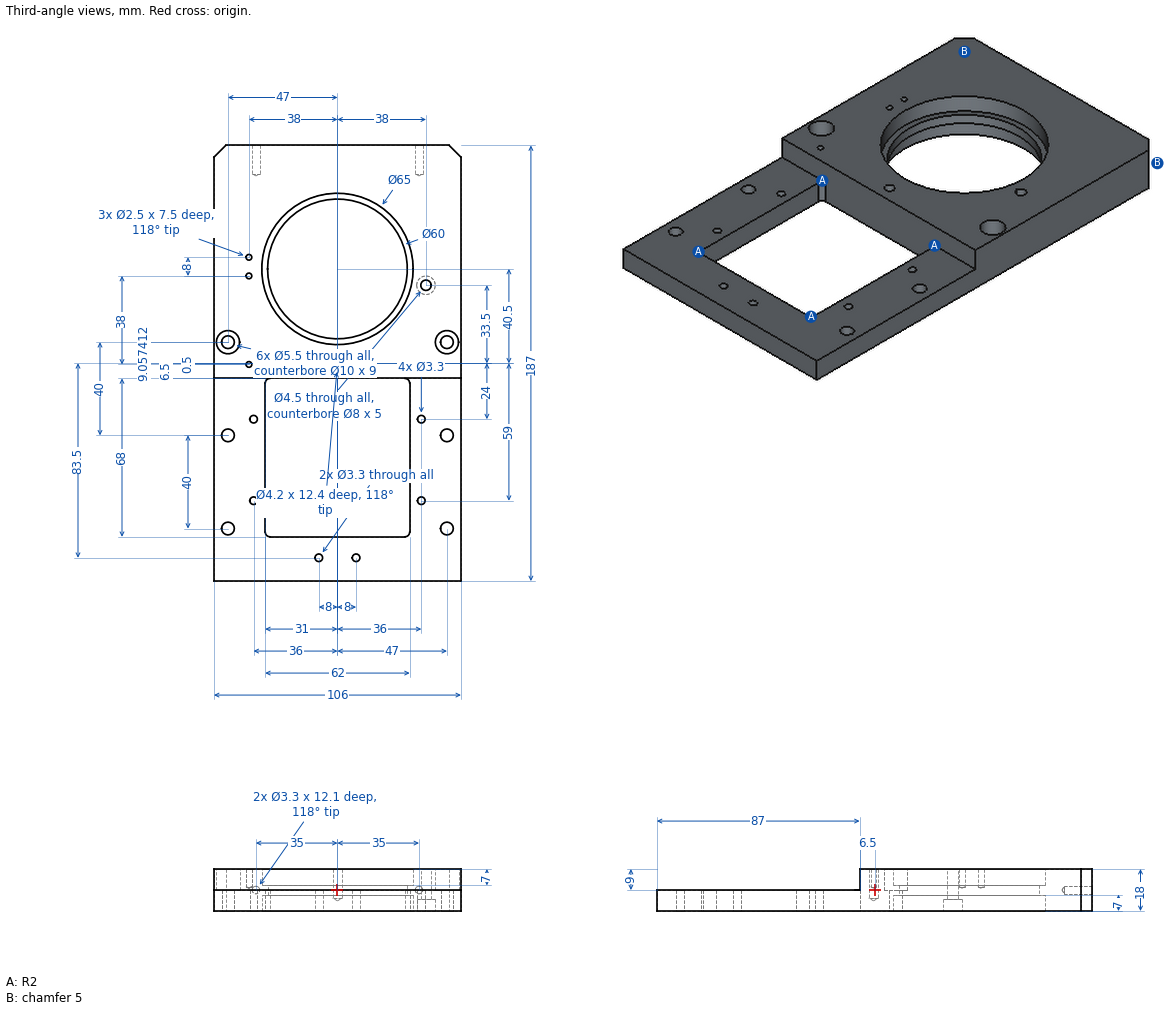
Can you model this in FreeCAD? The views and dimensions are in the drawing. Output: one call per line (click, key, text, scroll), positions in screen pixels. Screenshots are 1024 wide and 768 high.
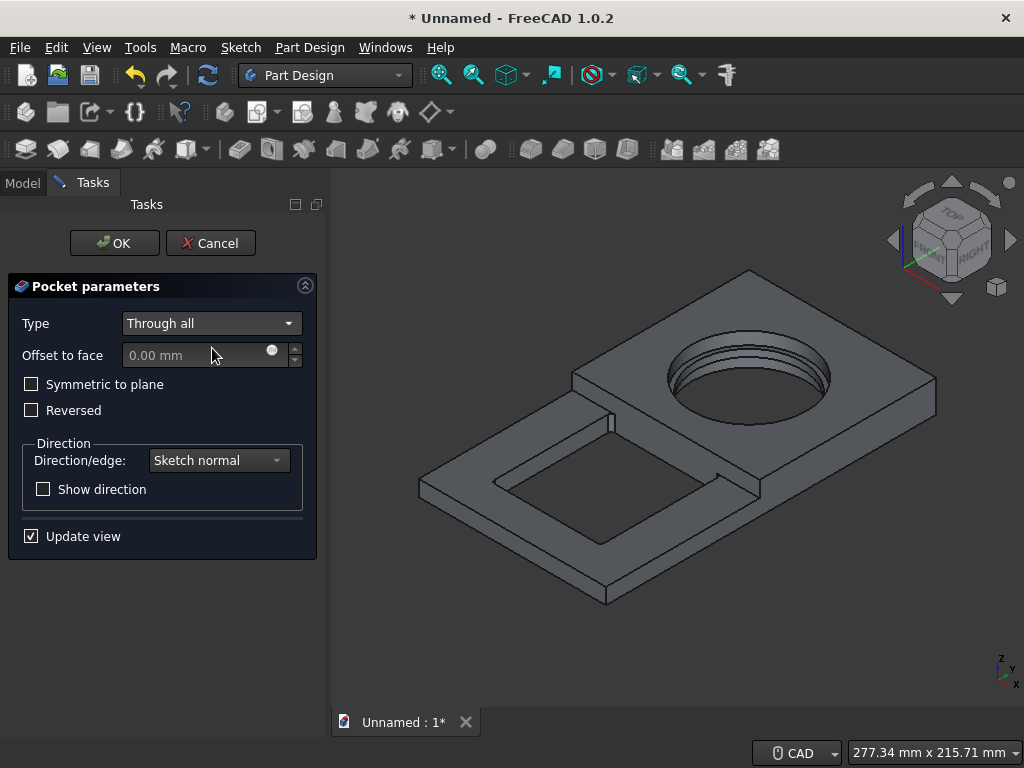
click(115, 243)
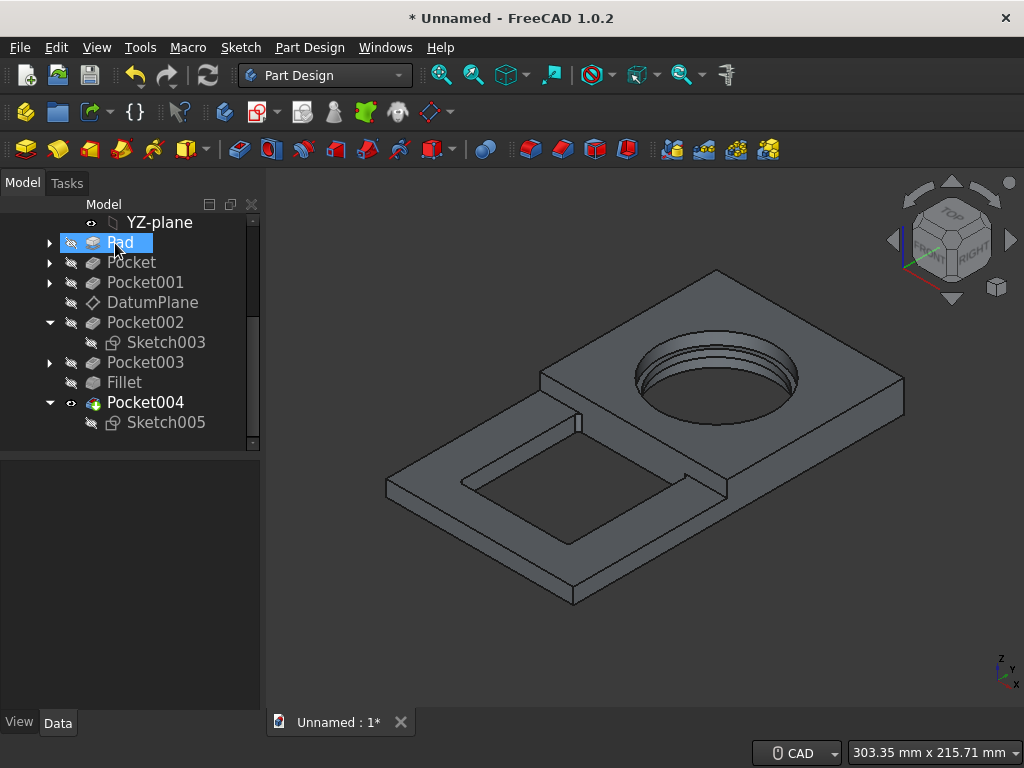
click(258, 112)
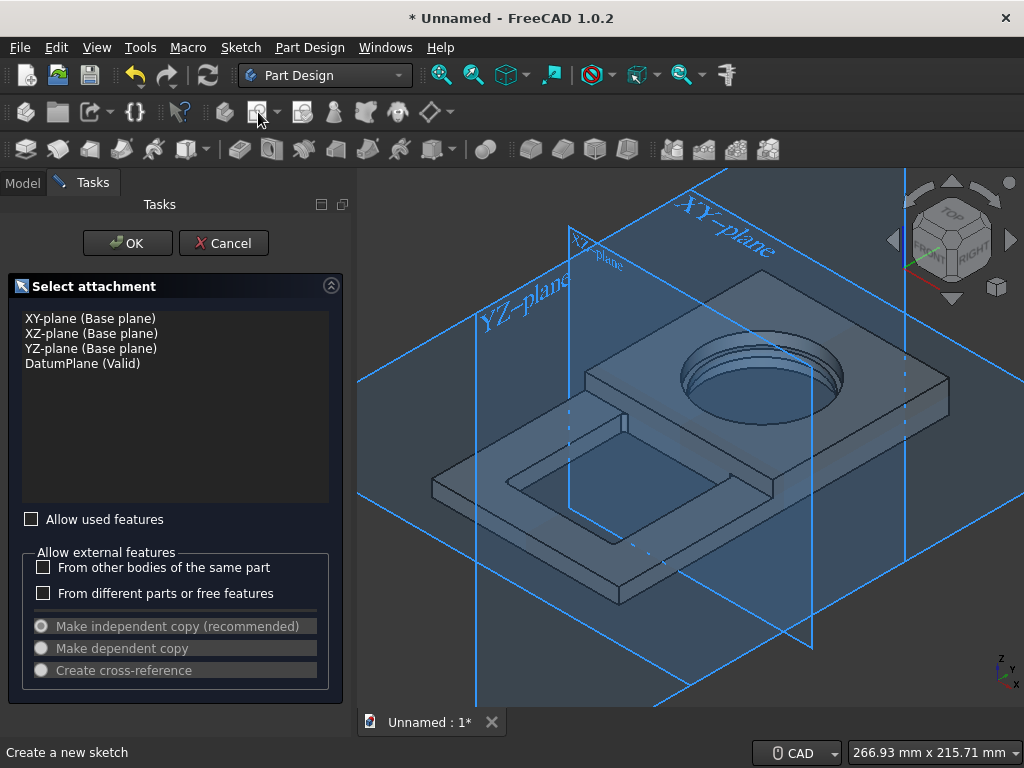
click(82, 318)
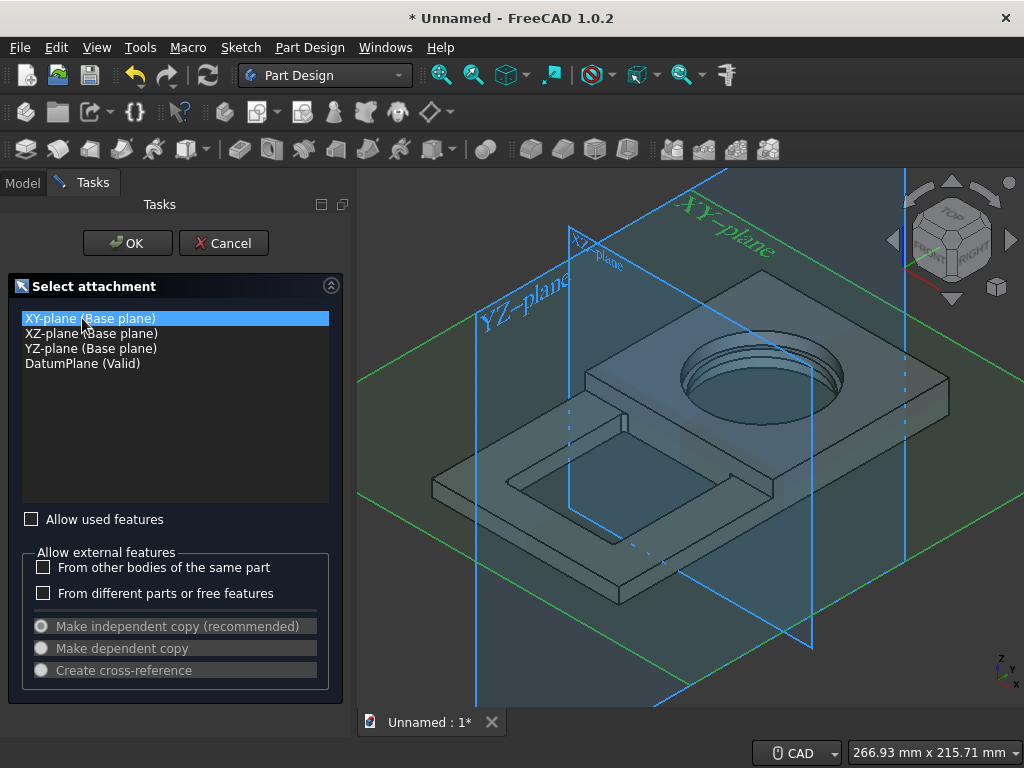
click(128, 243)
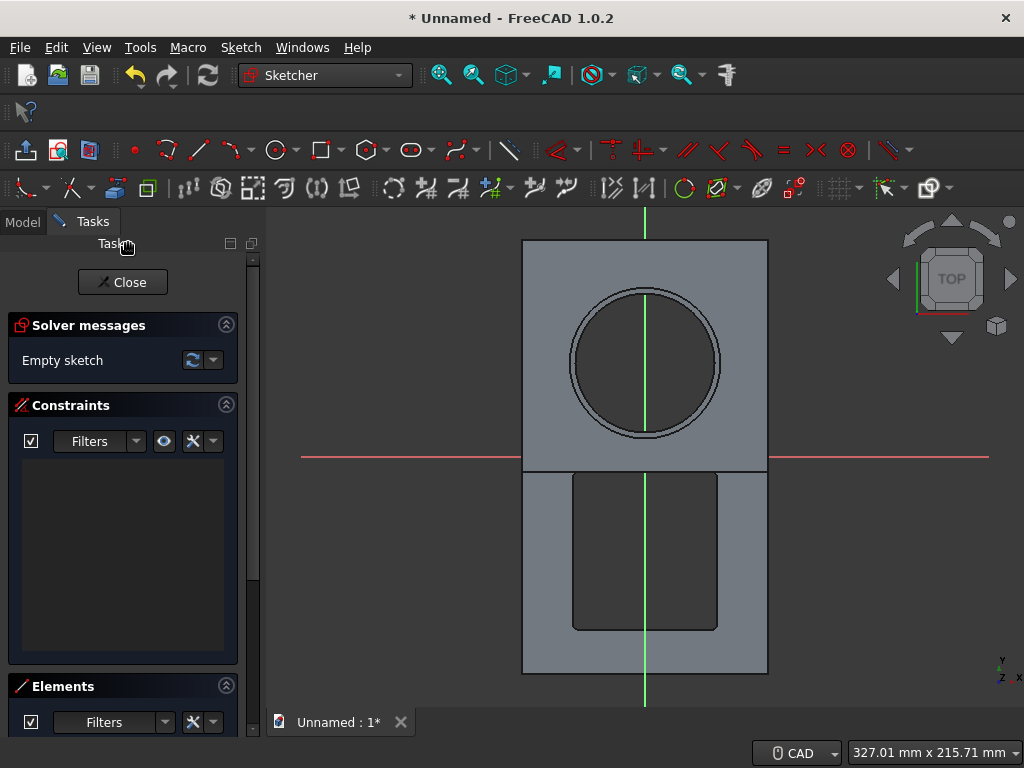
click(90, 150)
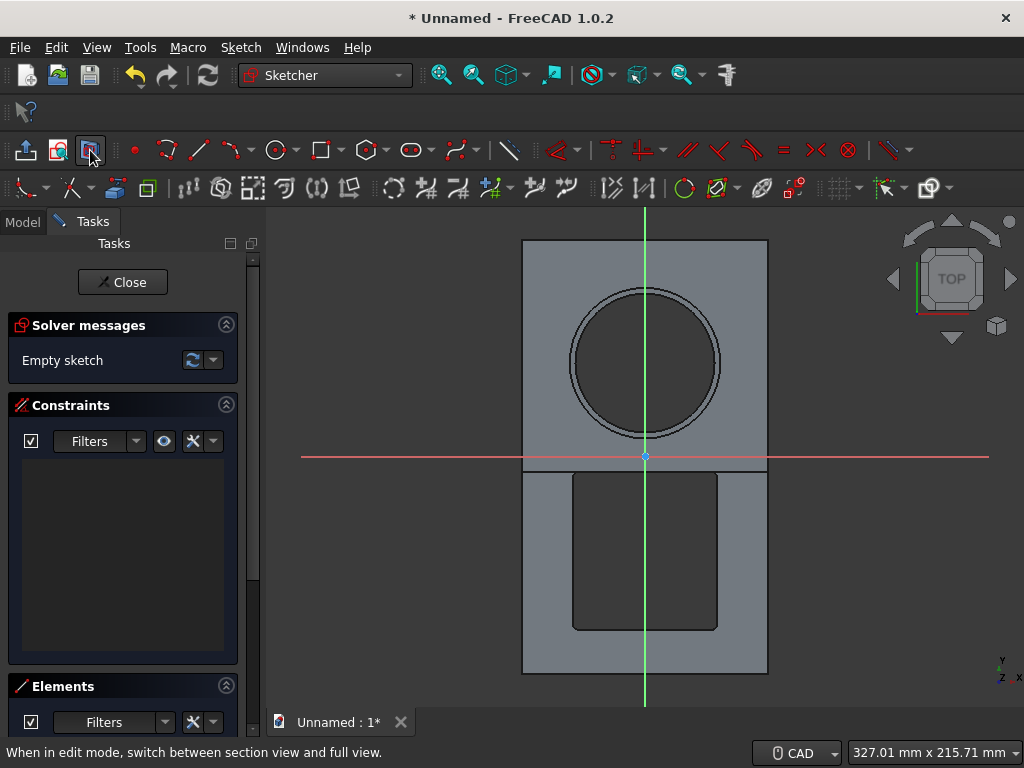
scroll(701, 585, up, 4)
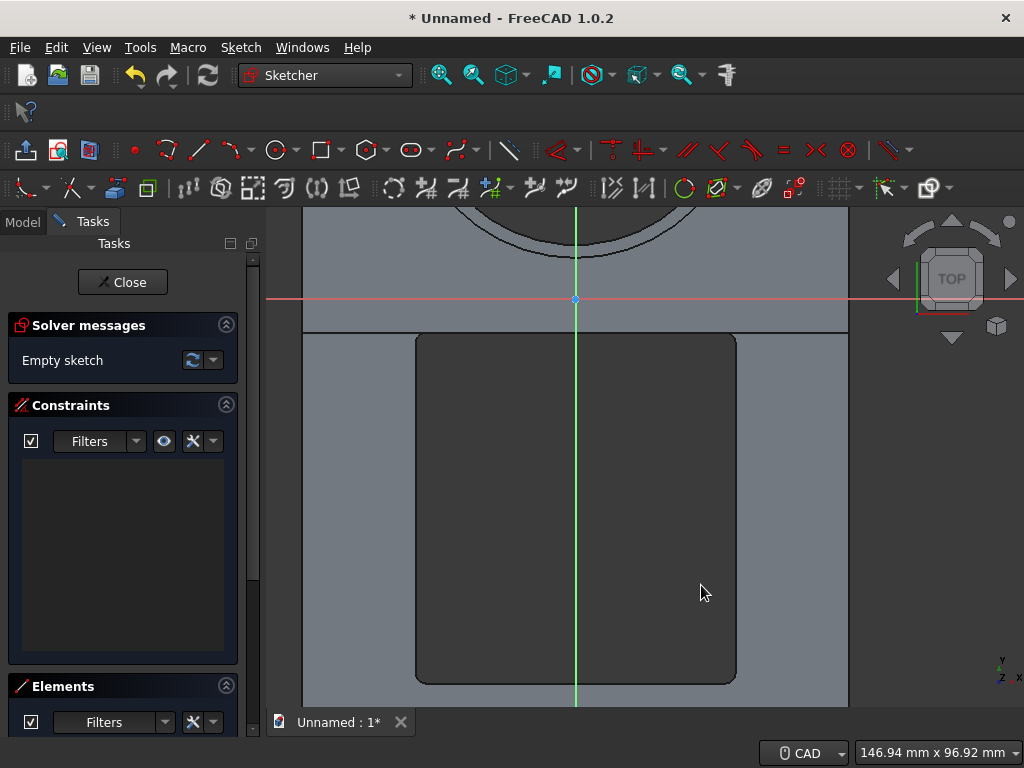
click(276, 150)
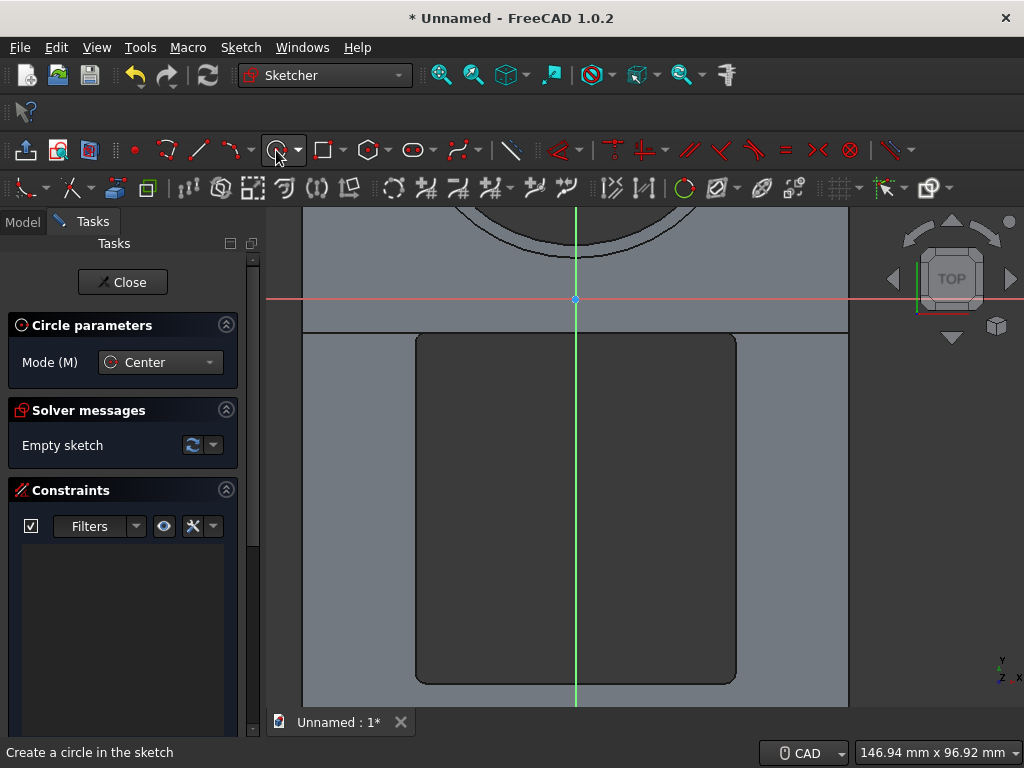
scroll(761, 423, up, 5)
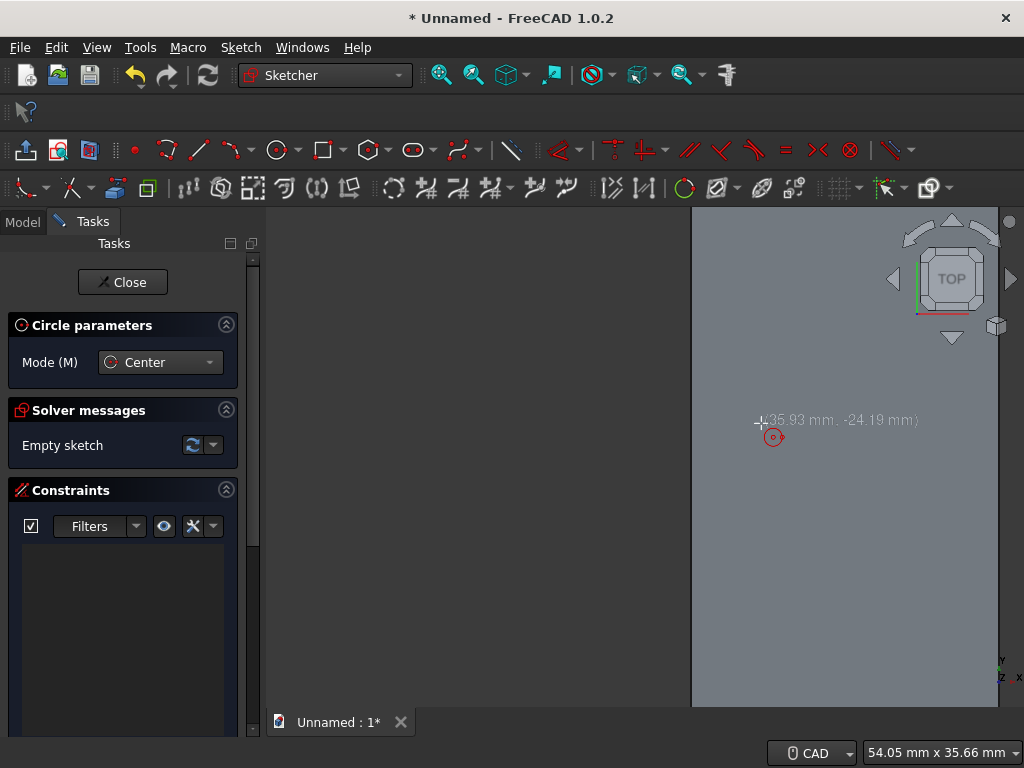
click(761, 422)
click(777, 406)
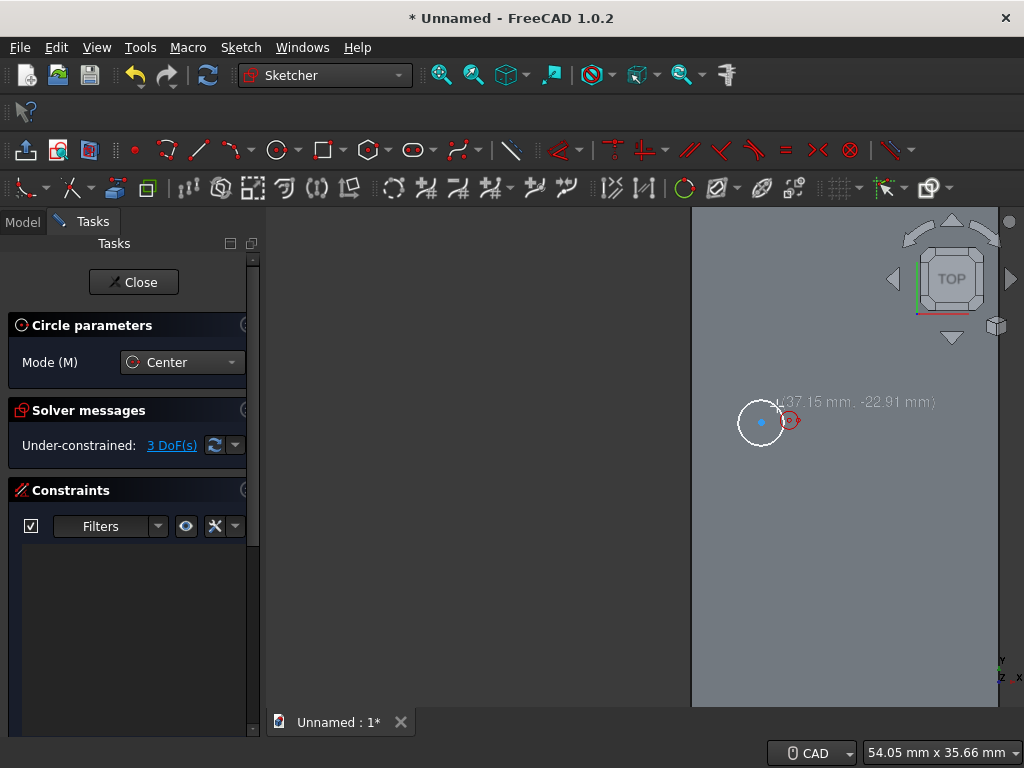
scroll(763, 426, down, 5)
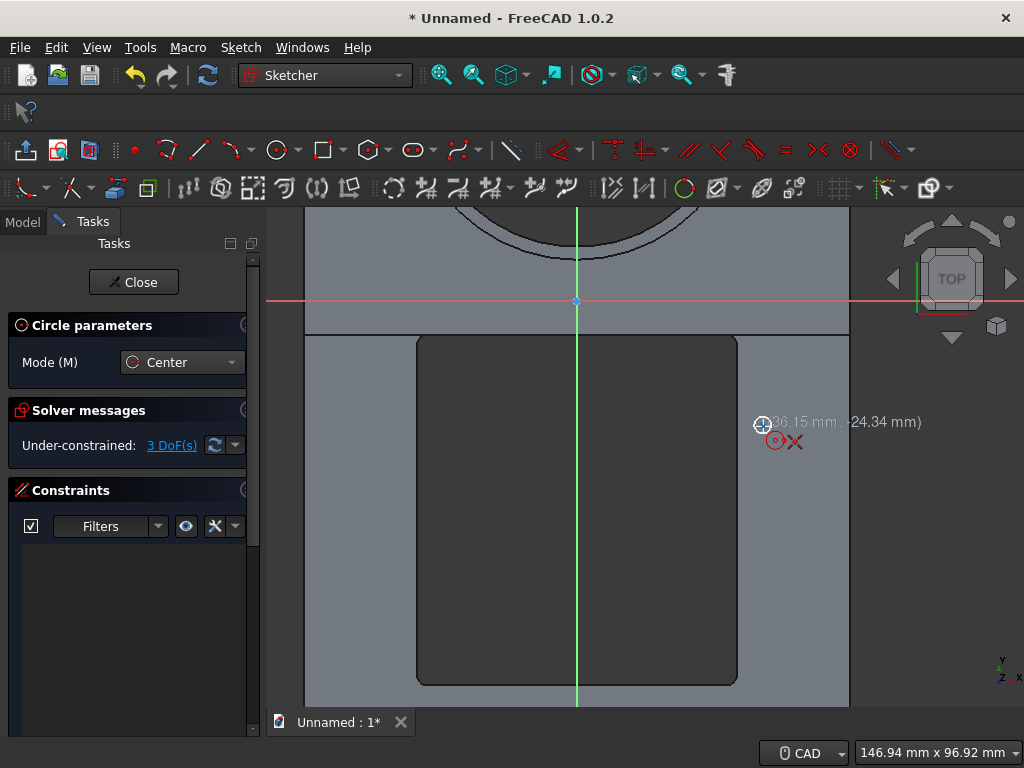
scroll(763, 605, up, 5)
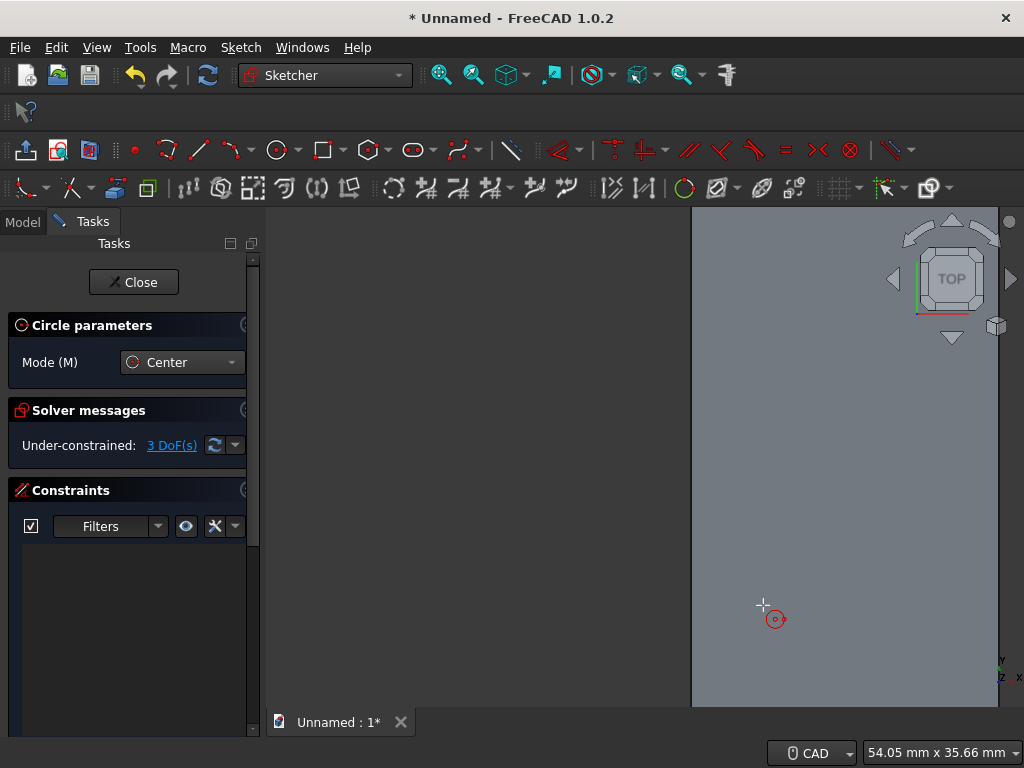
click(761, 605)
click(777, 589)